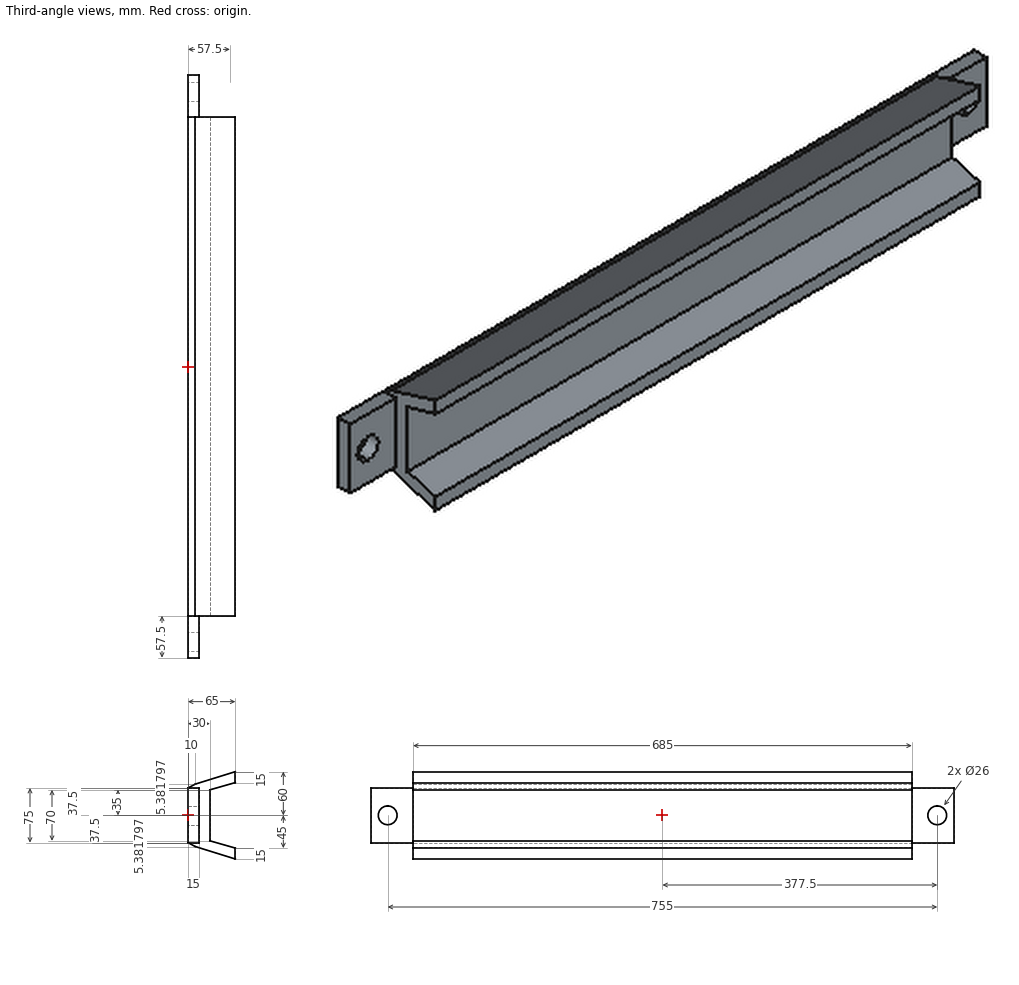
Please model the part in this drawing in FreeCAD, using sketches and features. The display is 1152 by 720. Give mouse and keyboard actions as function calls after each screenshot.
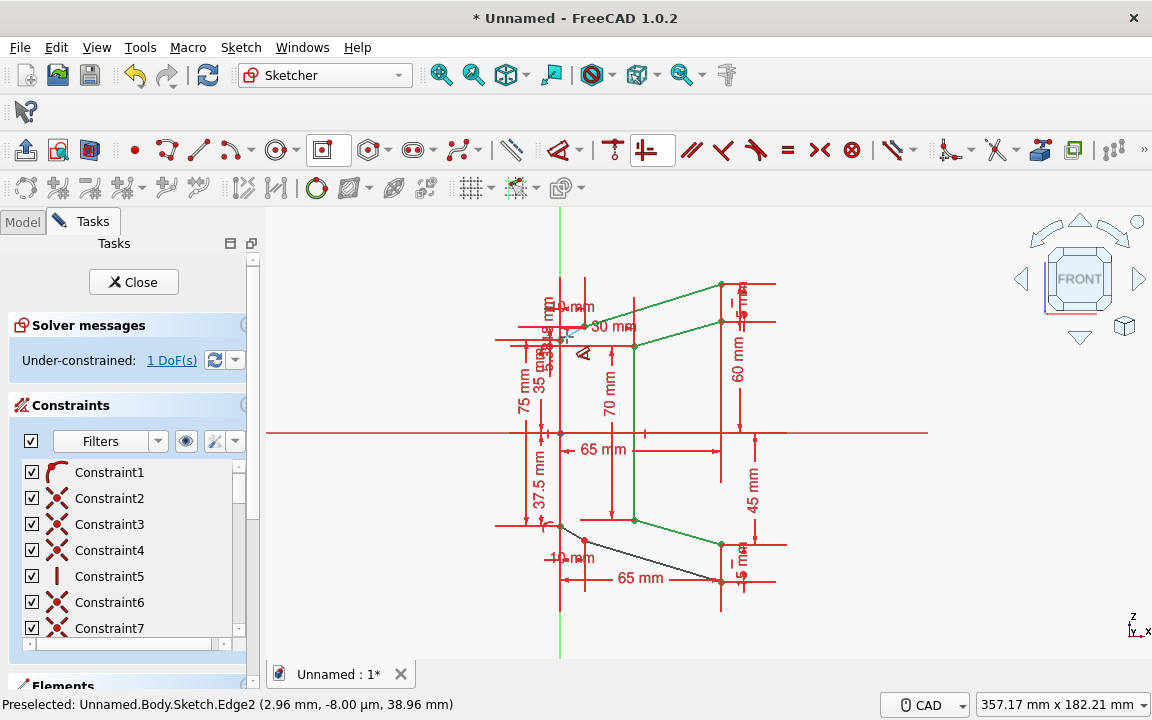
scroll(577, 537, up, 6)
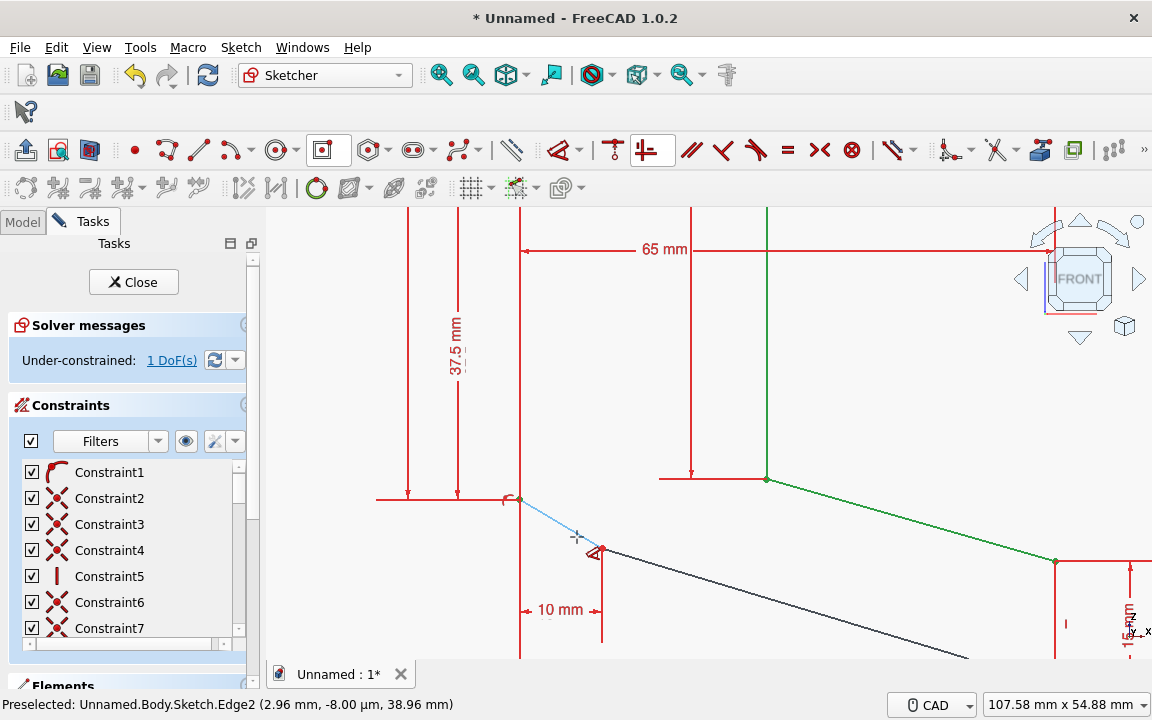
click(578, 534)
click(486, 524)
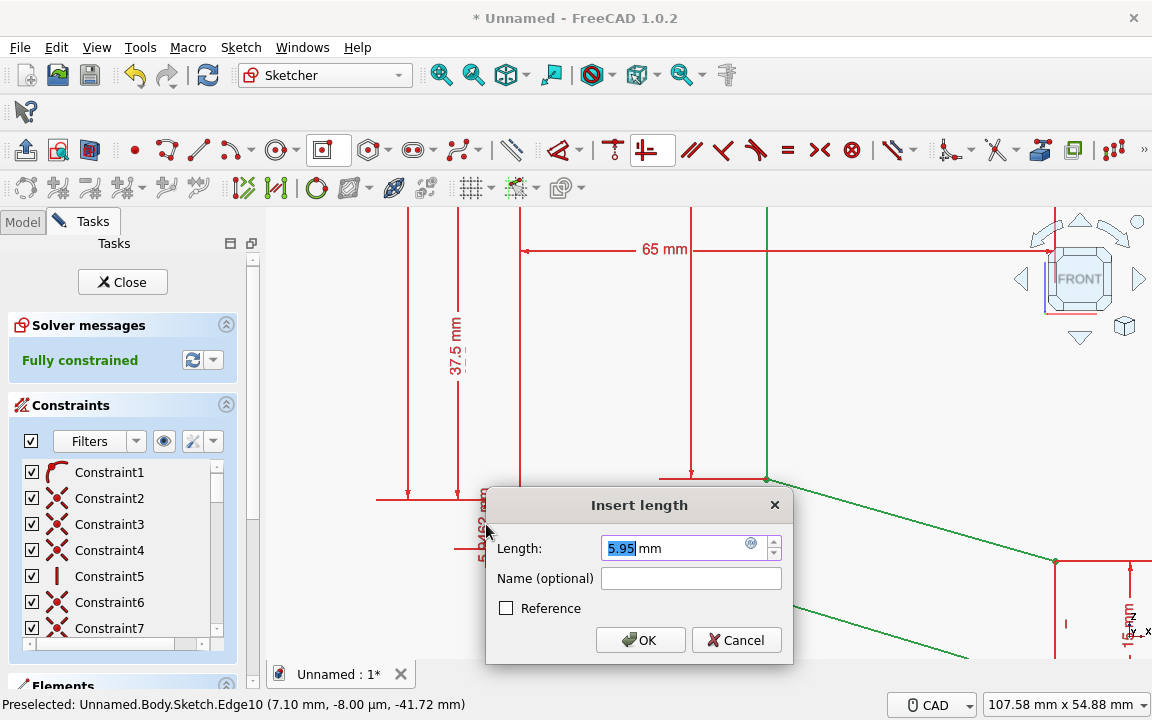
text(5.381797)
key(Return)
key(Escape)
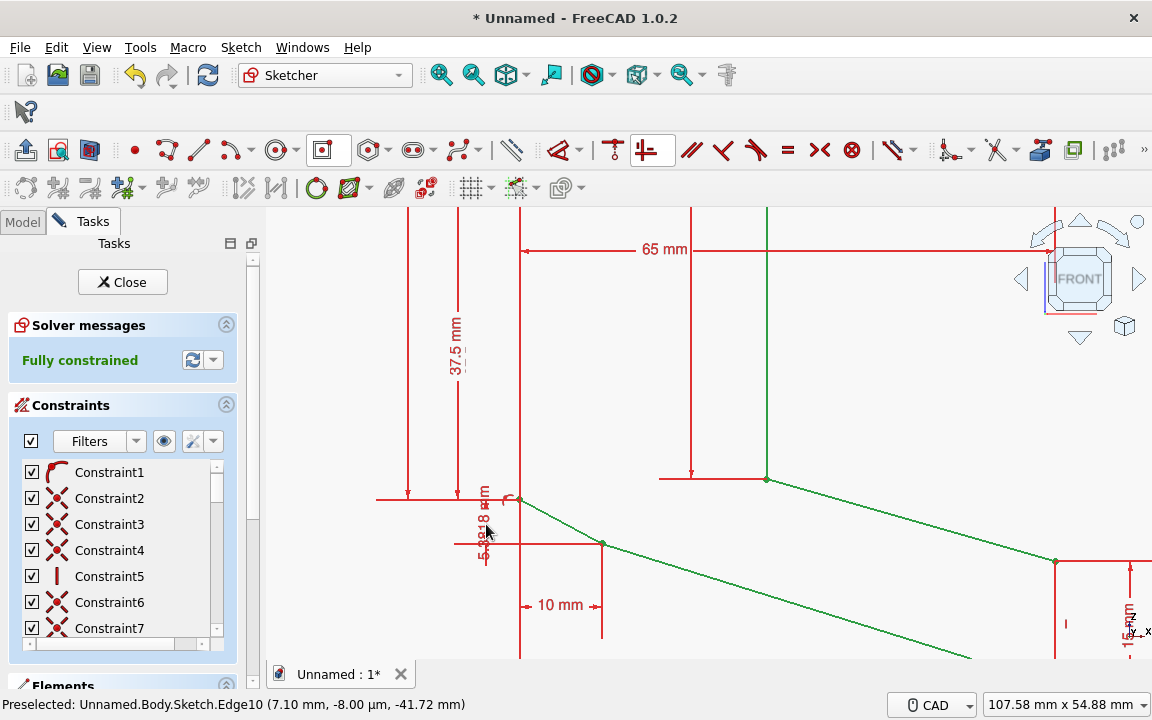
click(123, 282)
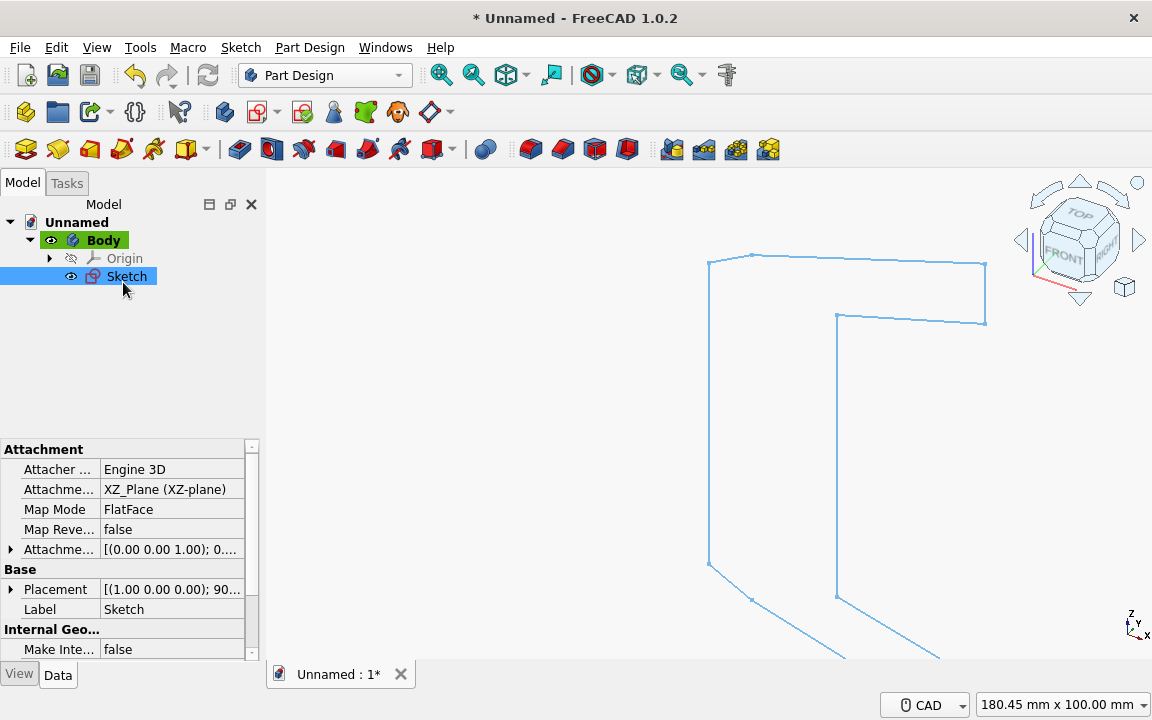
click(26, 150)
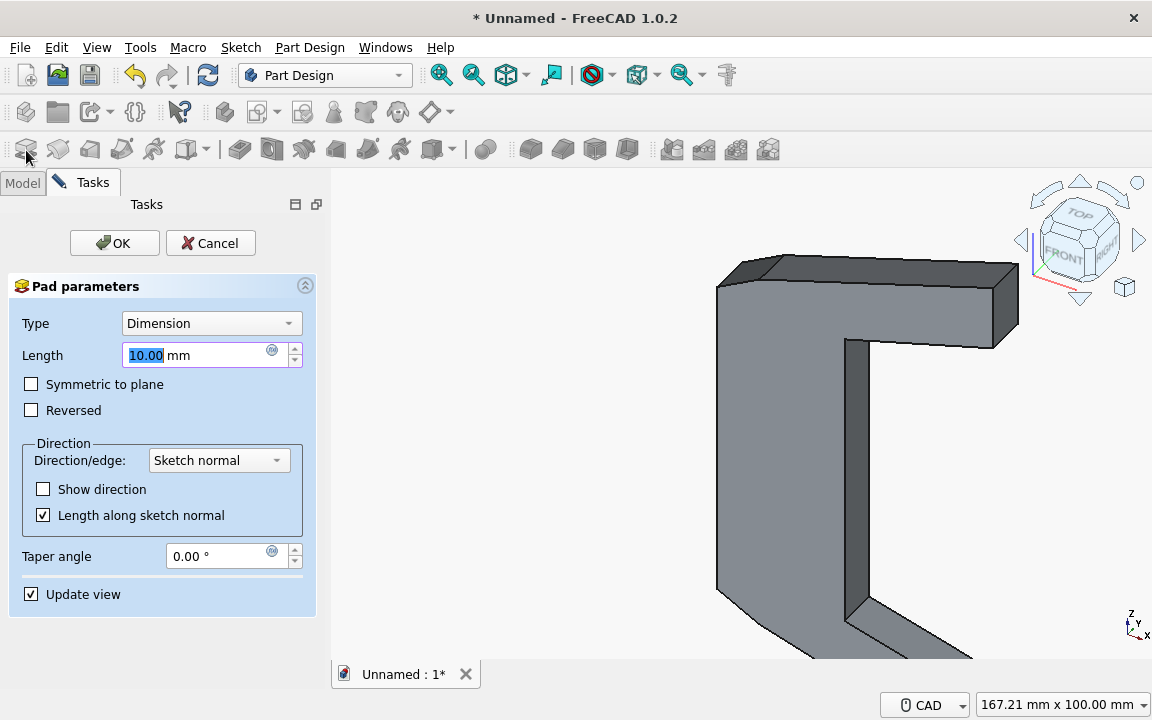
text(685)
key(Tab)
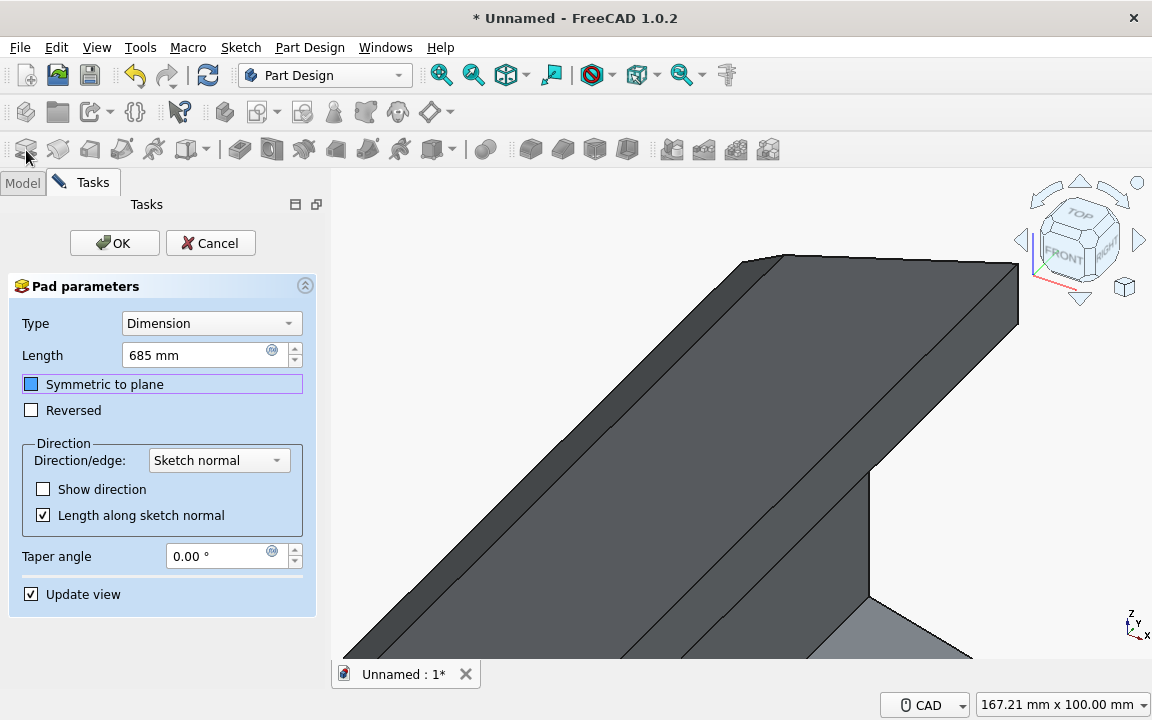
click(30, 384)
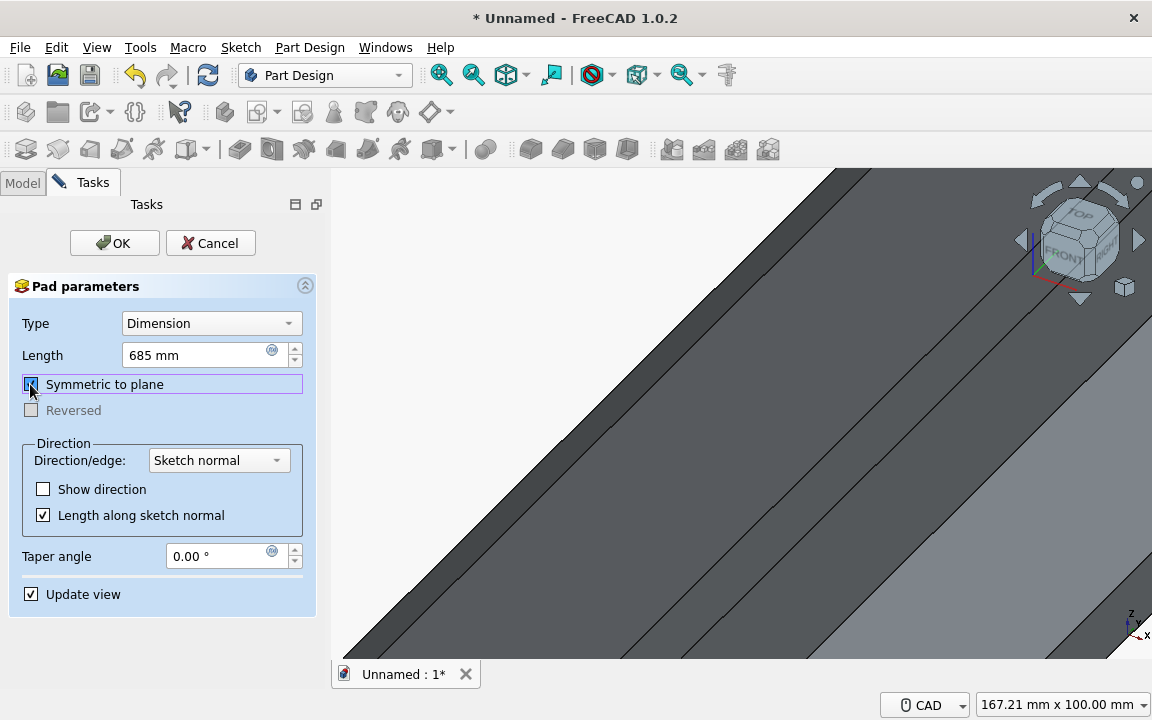
click(115, 243)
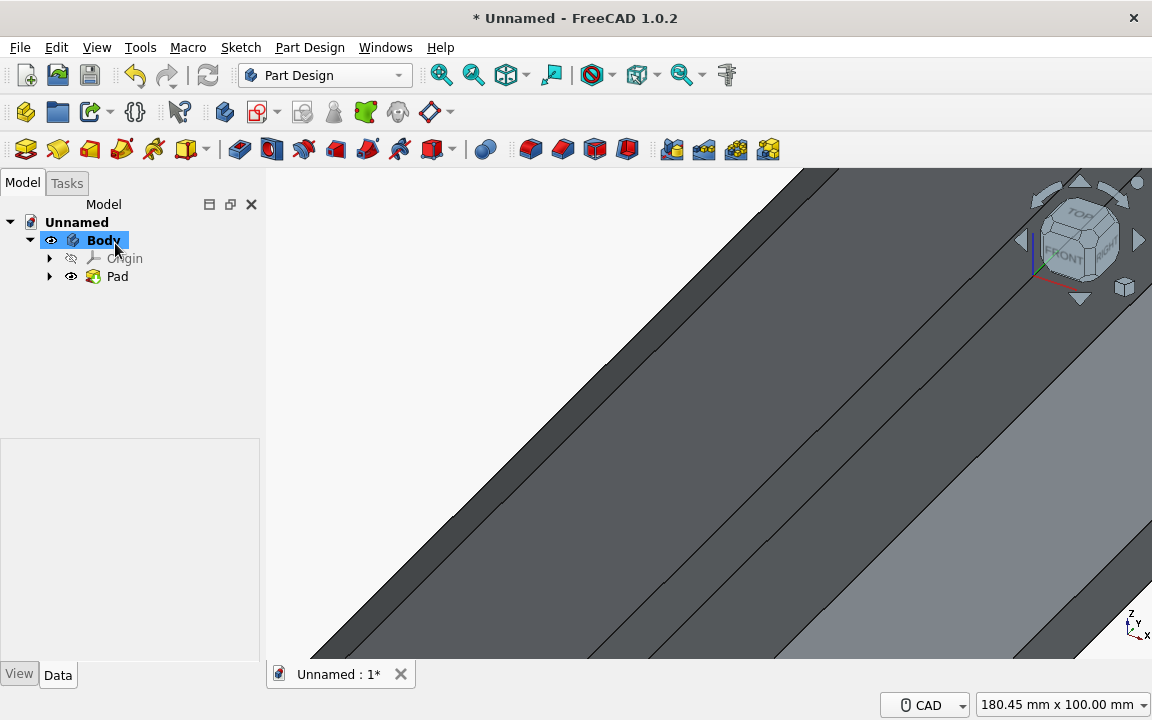
click(442, 76)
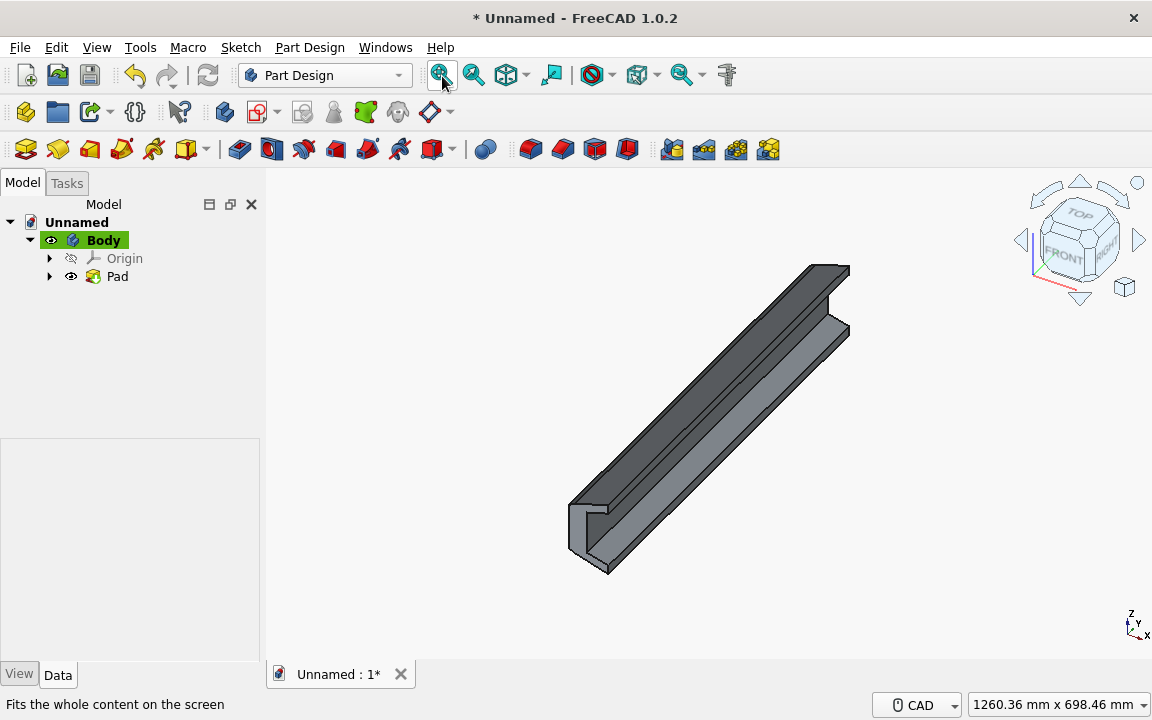
click(577, 518)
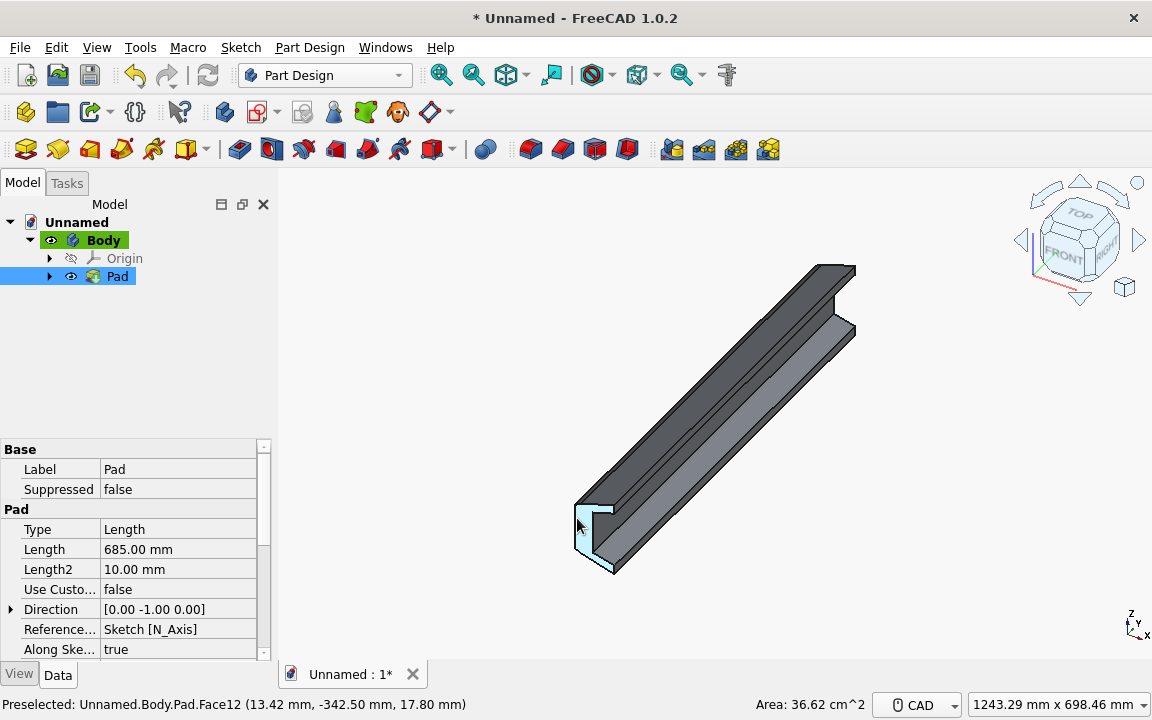
click(258, 112)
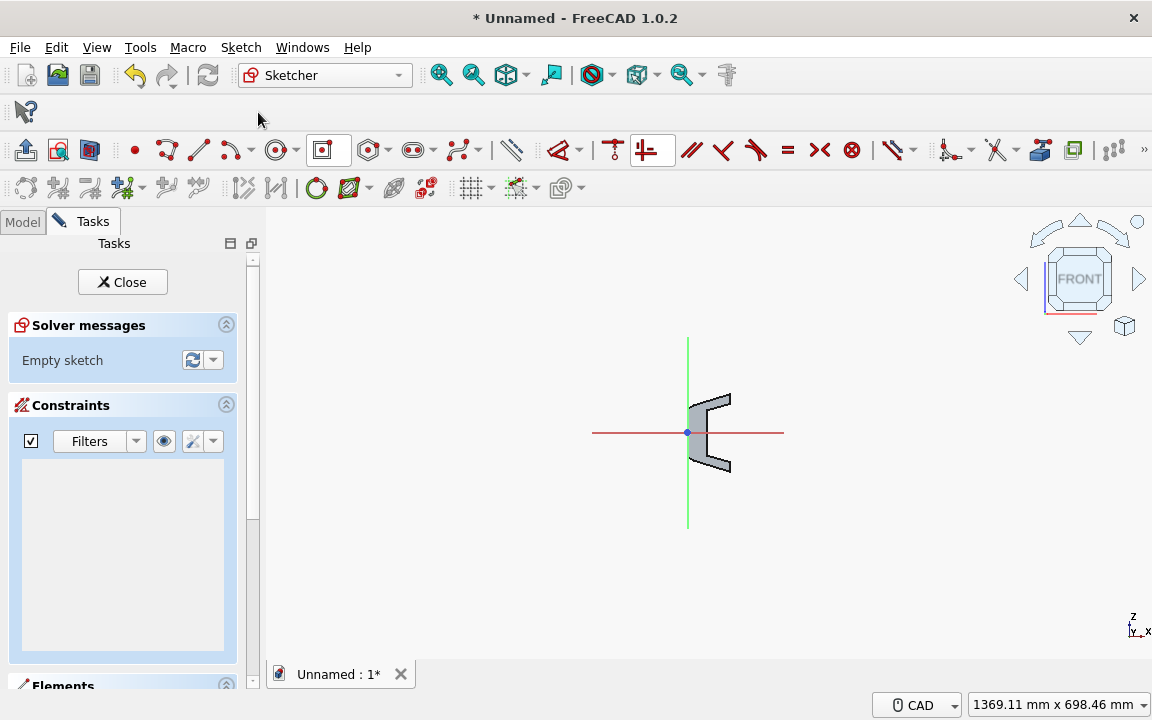
scroll(703, 433, up, 9)